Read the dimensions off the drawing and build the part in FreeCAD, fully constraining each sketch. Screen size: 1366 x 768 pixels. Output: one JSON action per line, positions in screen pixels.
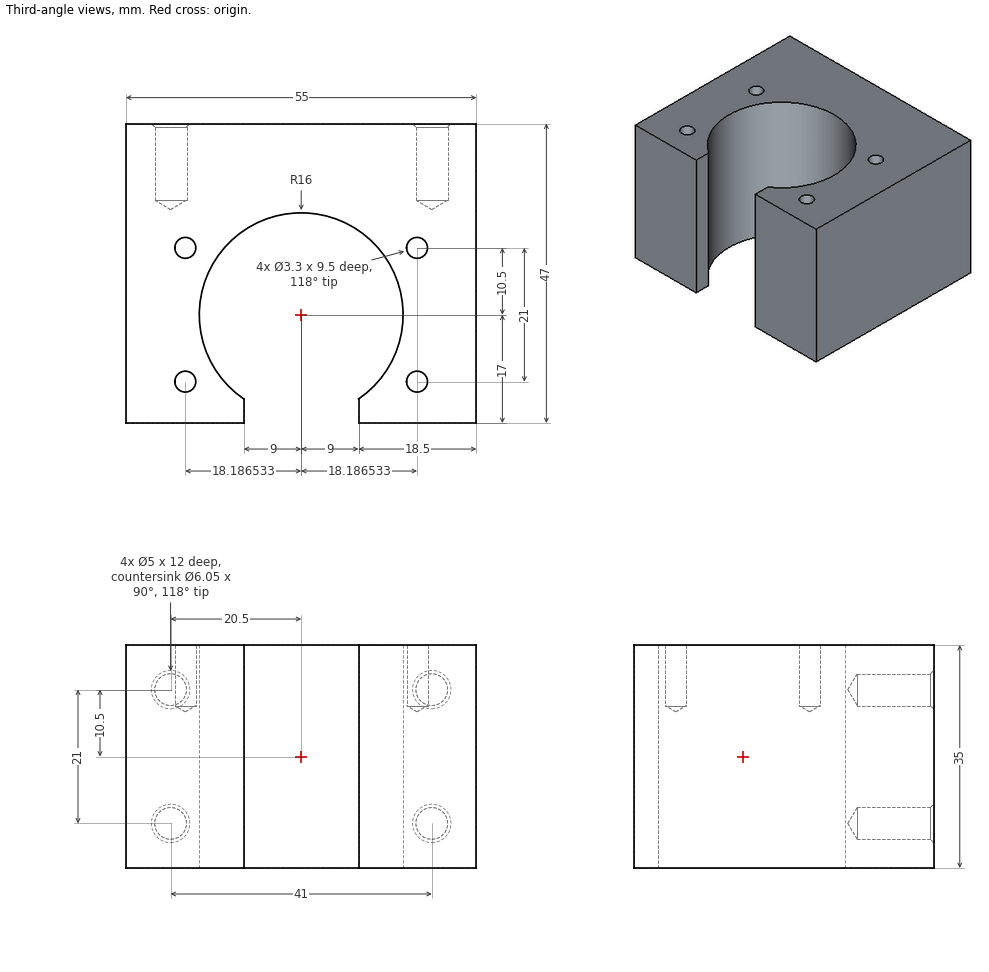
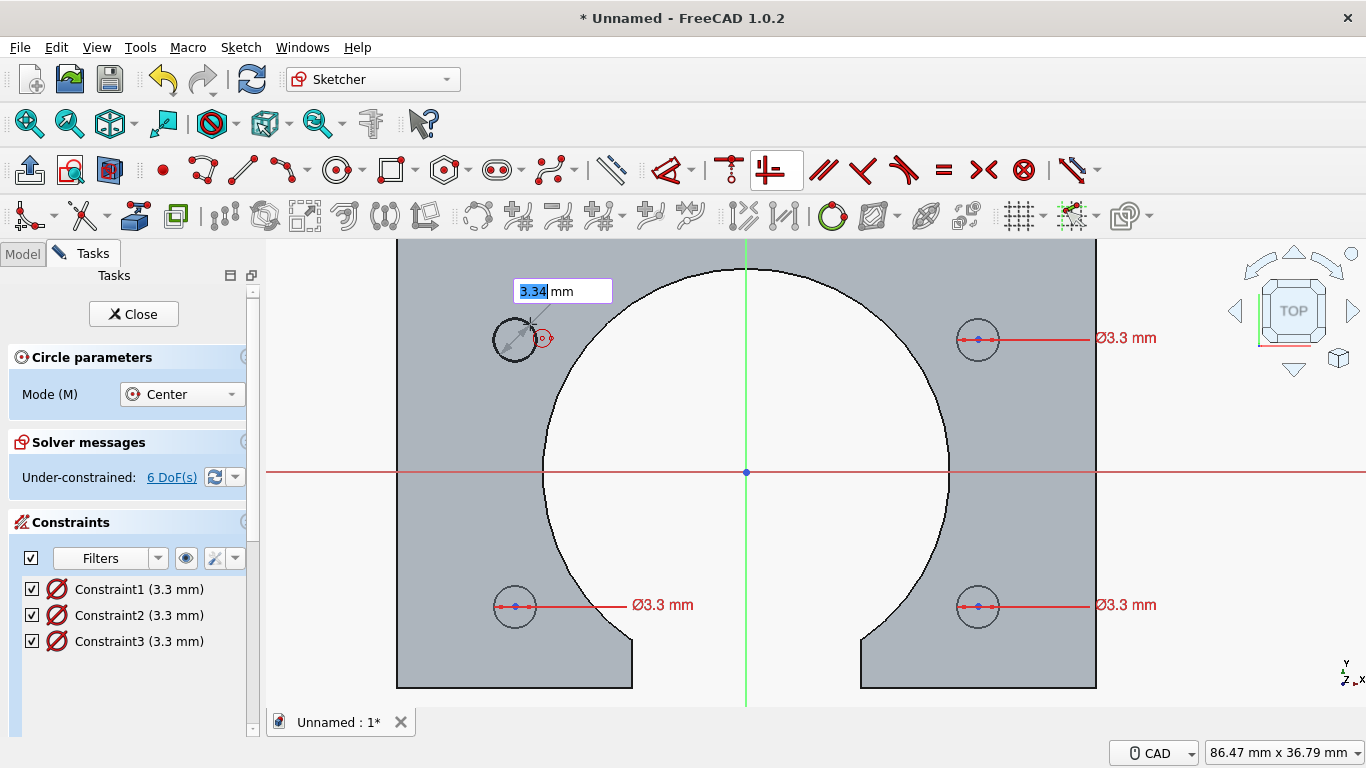
{"action": "type", "text": "3.3"}
{"action": "key", "text": "Return"}
{"action": "key", "text": "Escape"}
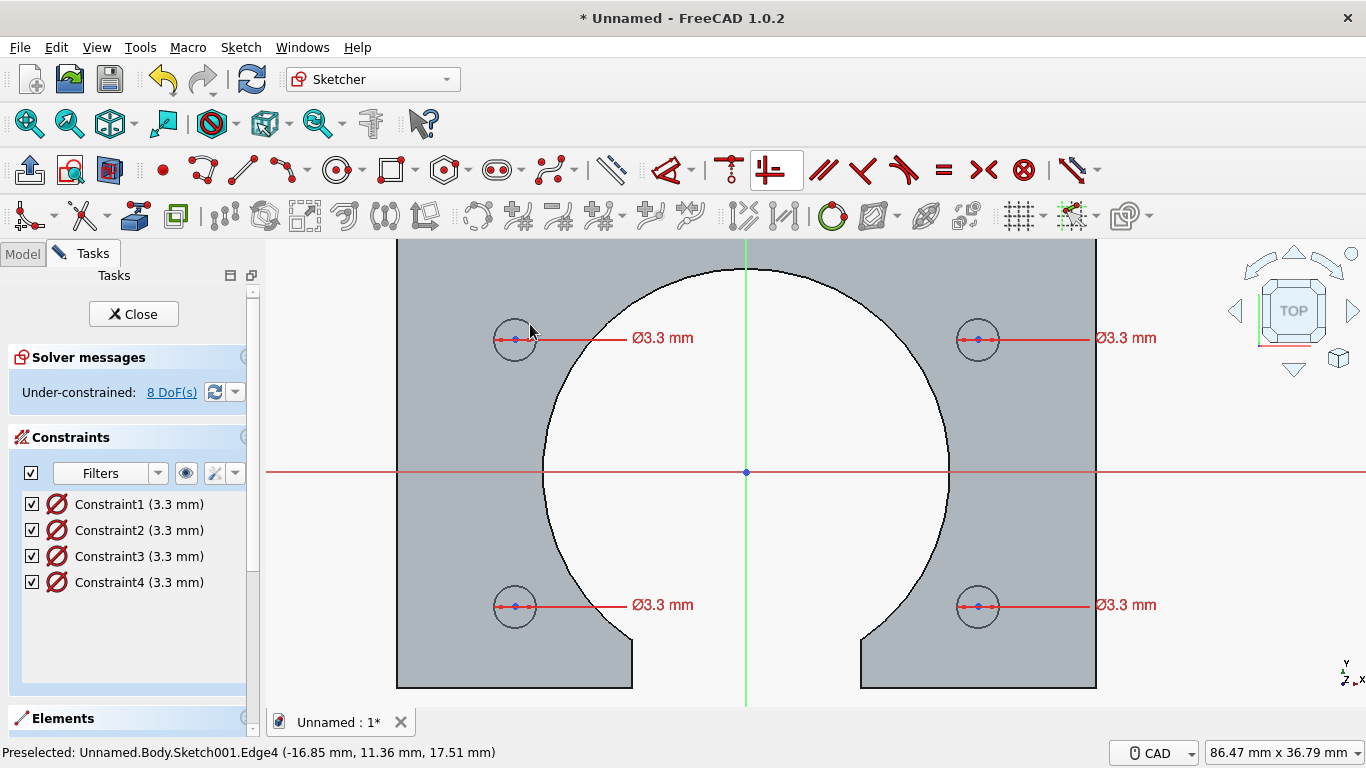
{"action": "left_click", "coordinate": [666, 170]}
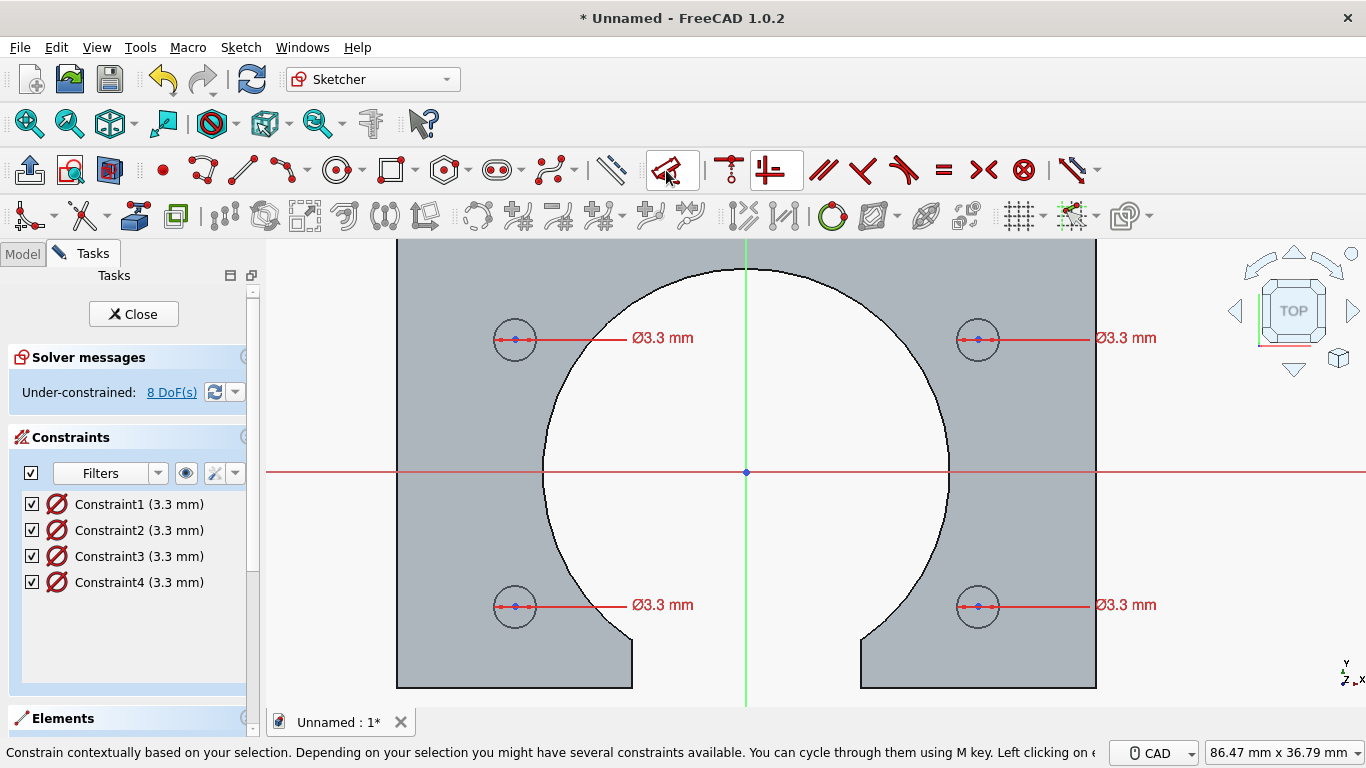
{"action": "left_click", "coordinate": [978, 340]}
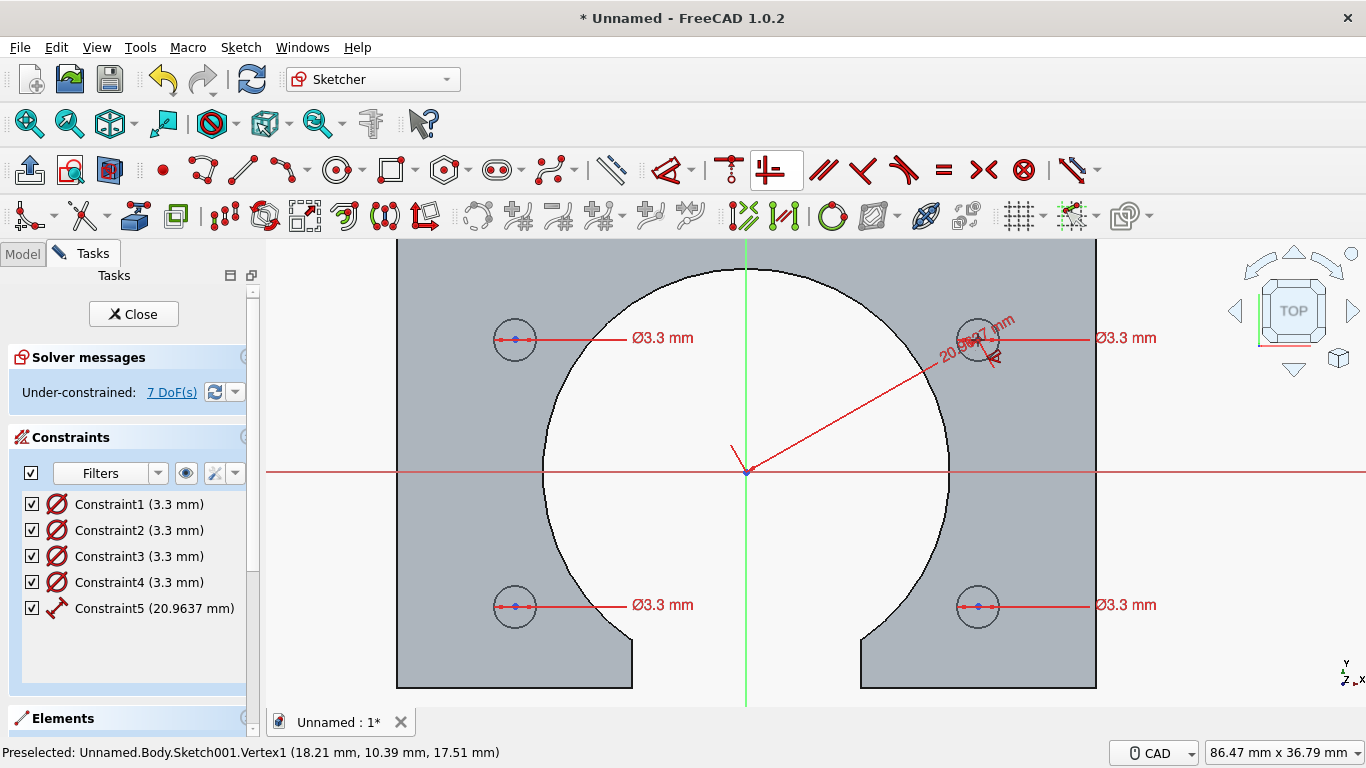
{"action": "left_click", "coordinate": [978, 607]}
{"action": "left_click", "coordinate": [1012, 412]}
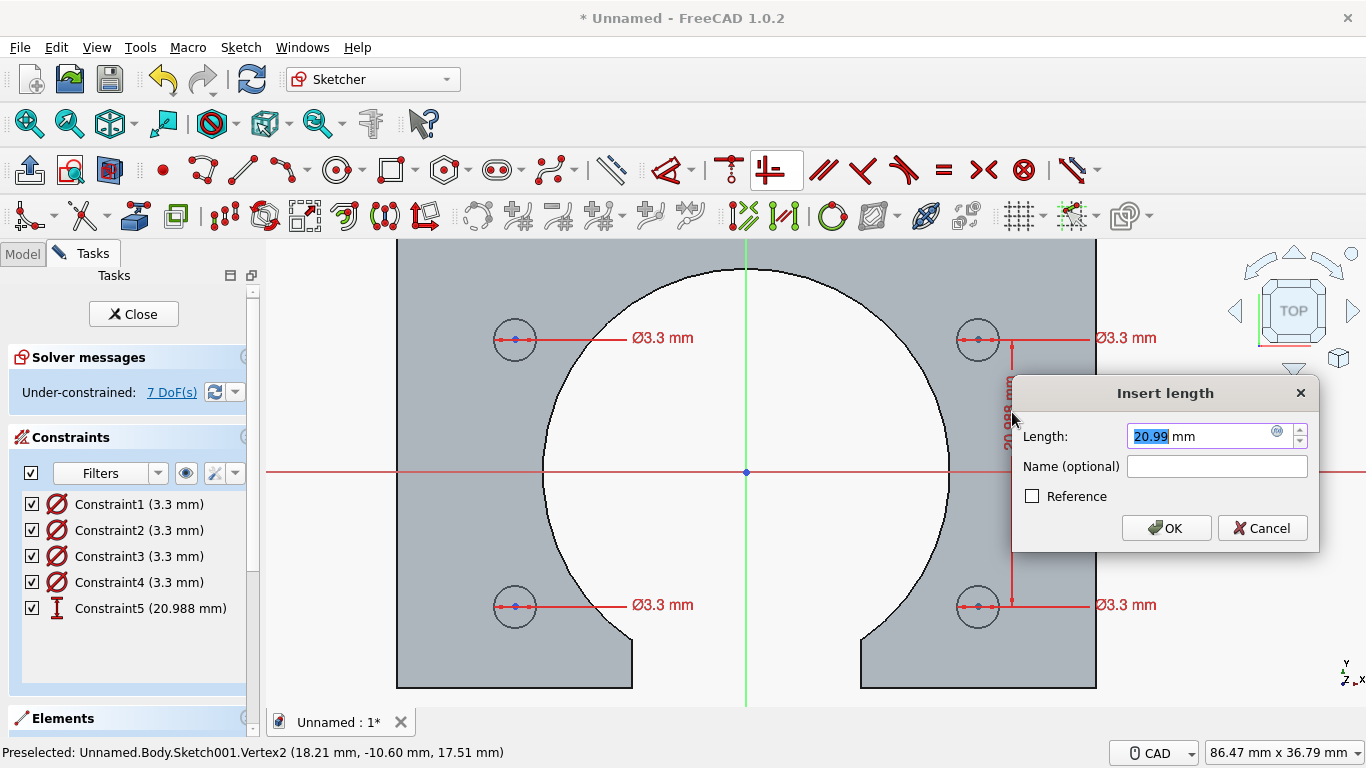
{"action": "type", "text": "21"}
{"action": "key", "text": "Return"}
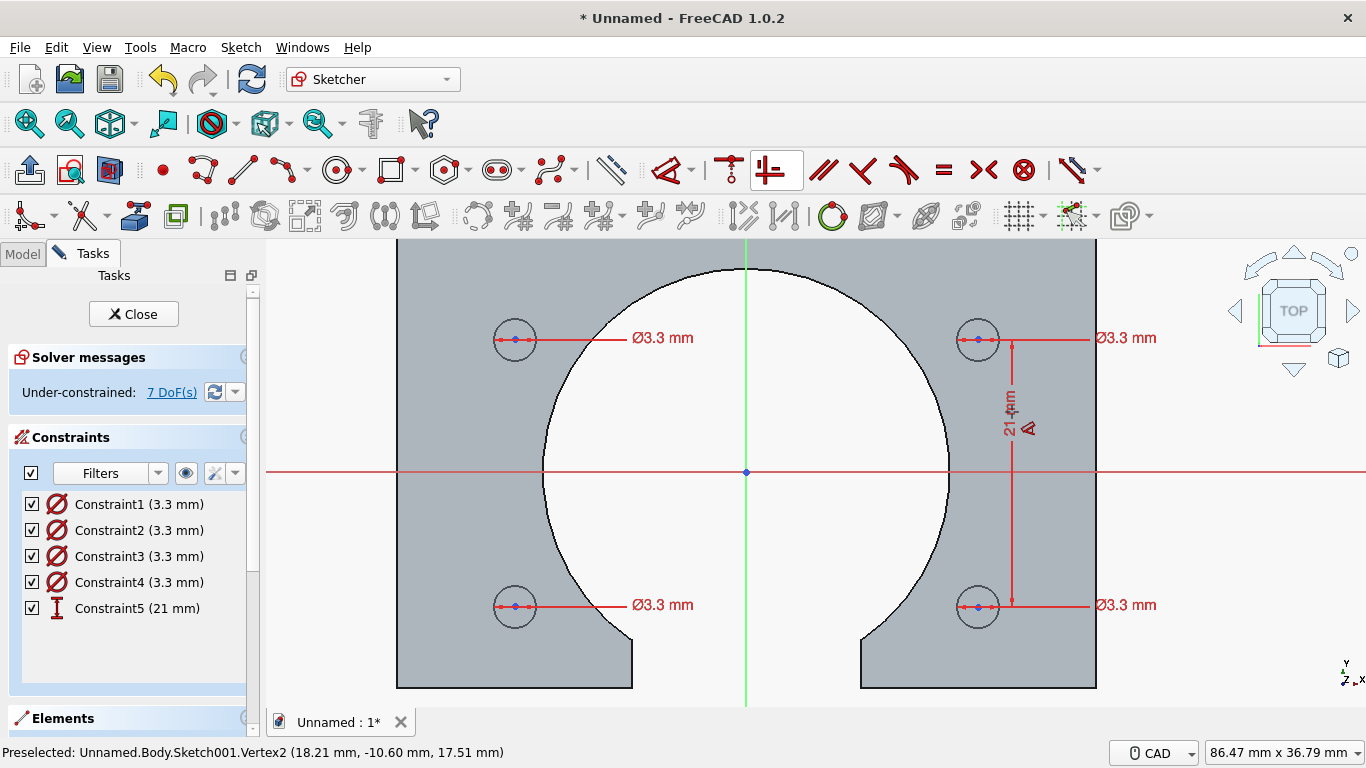
{"action": "left_click", "coordinate": [978, 340]}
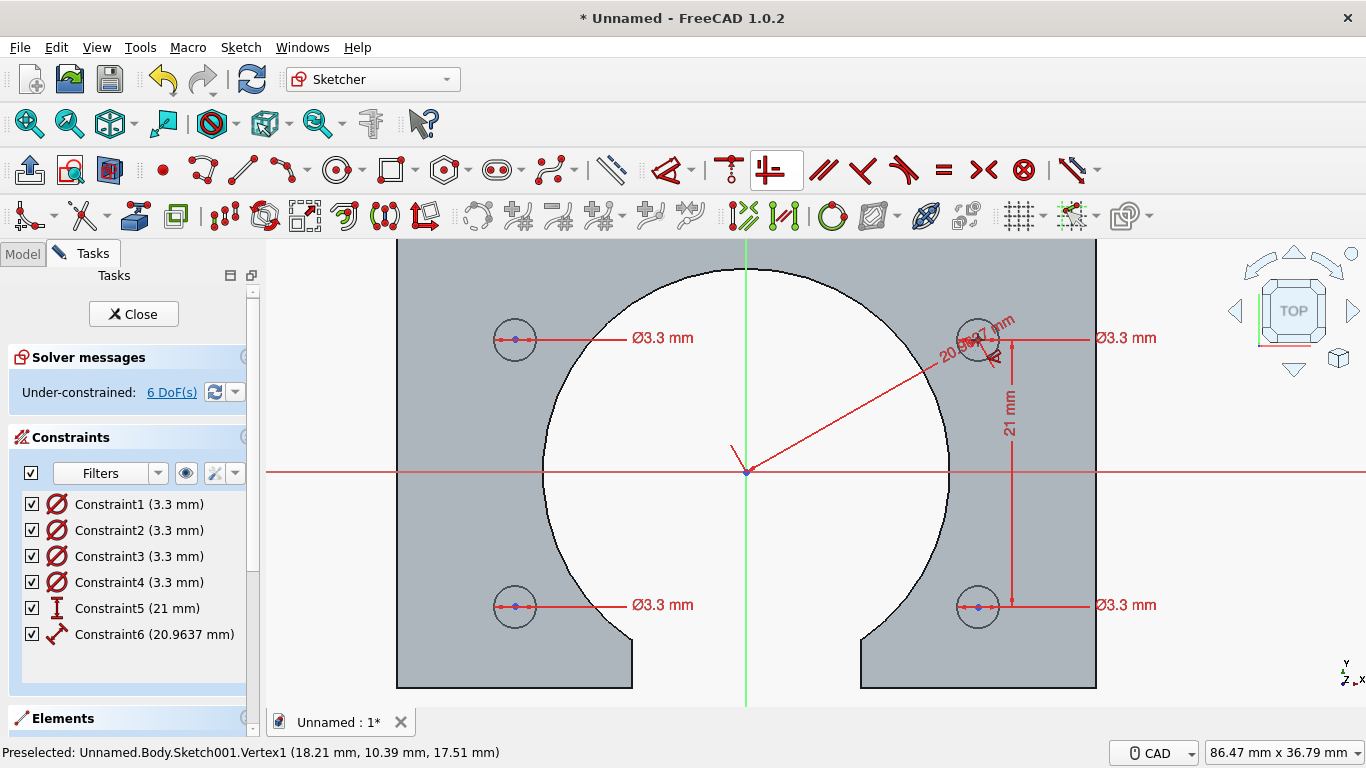
{"action": "left_click", "coordinate": [515, 607]}
{"action": "left_click", "coordinate": [1012, 535]}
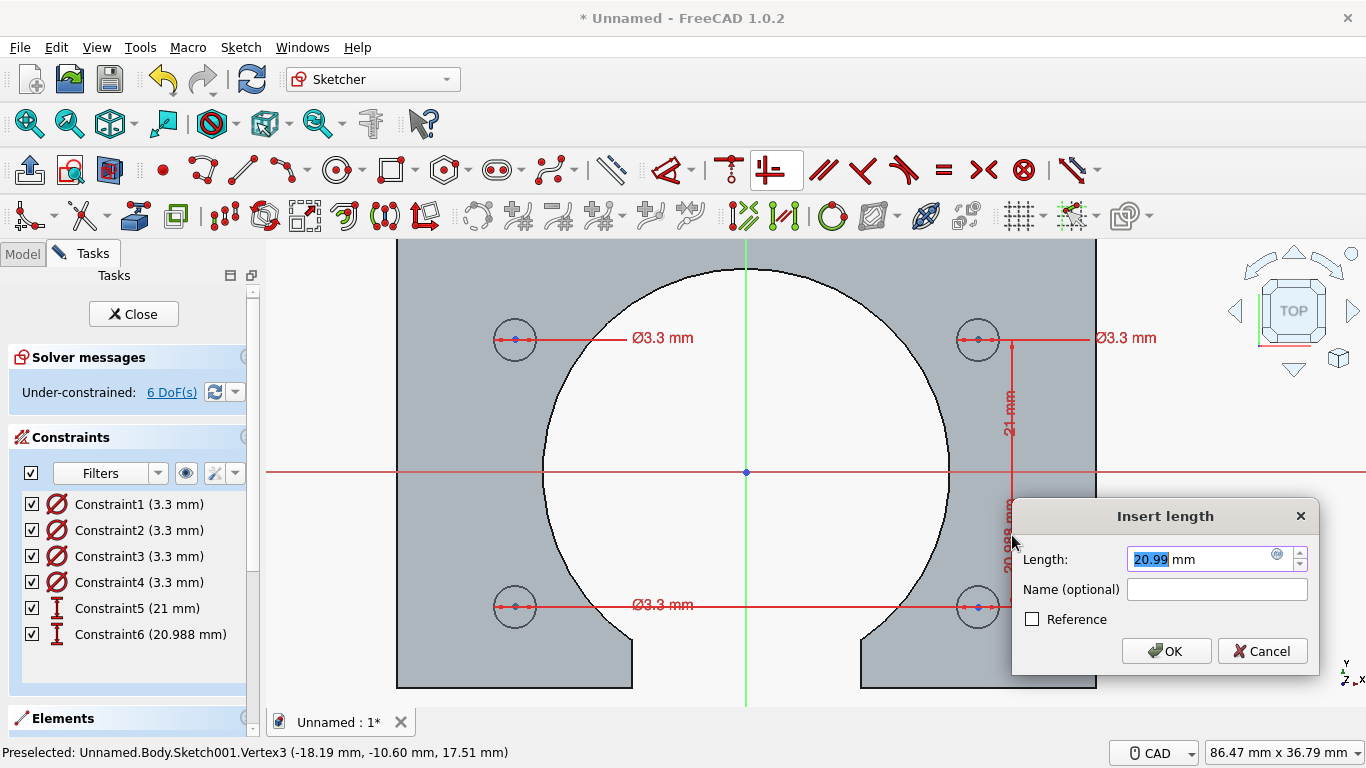
{"action": "type", "text": "21"}
{"action": "key", "text": "Return"}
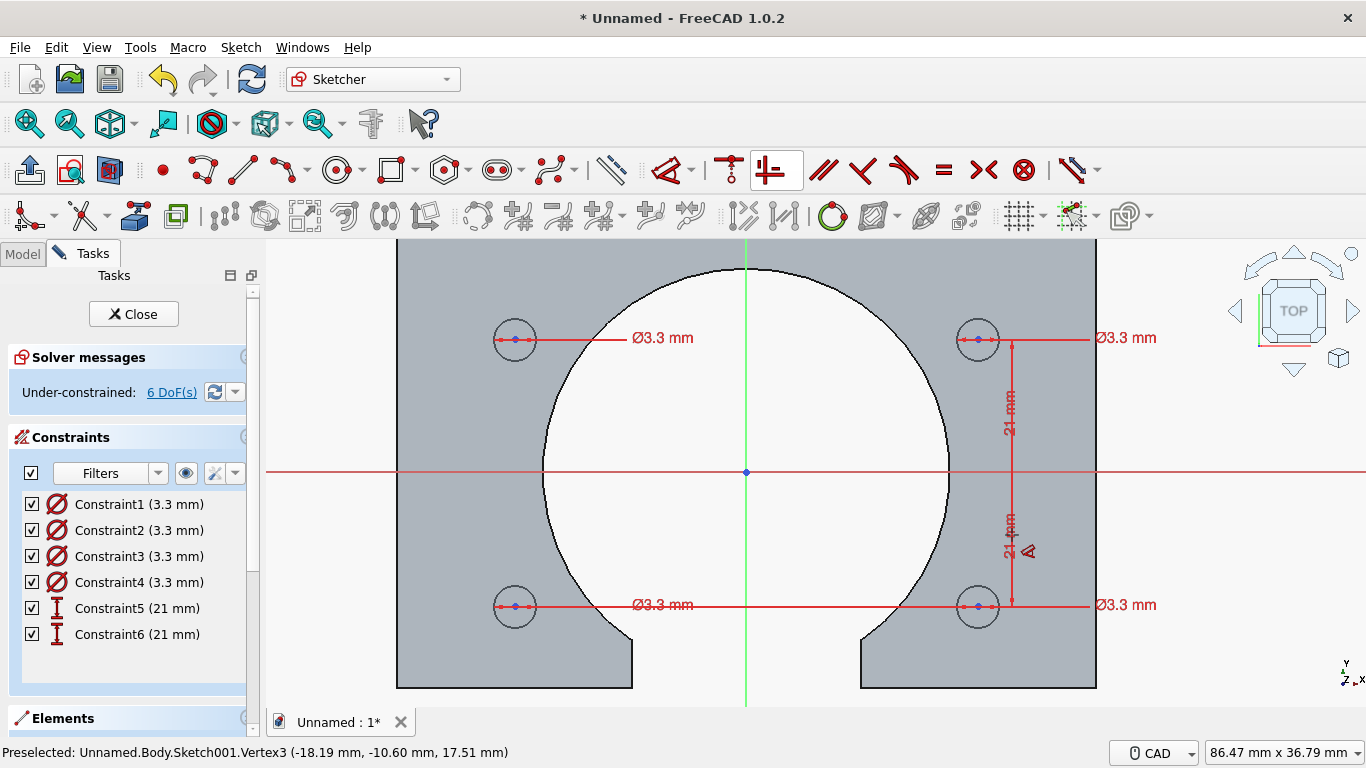
{"action": "left_click", "coordinate": [515, 607]}